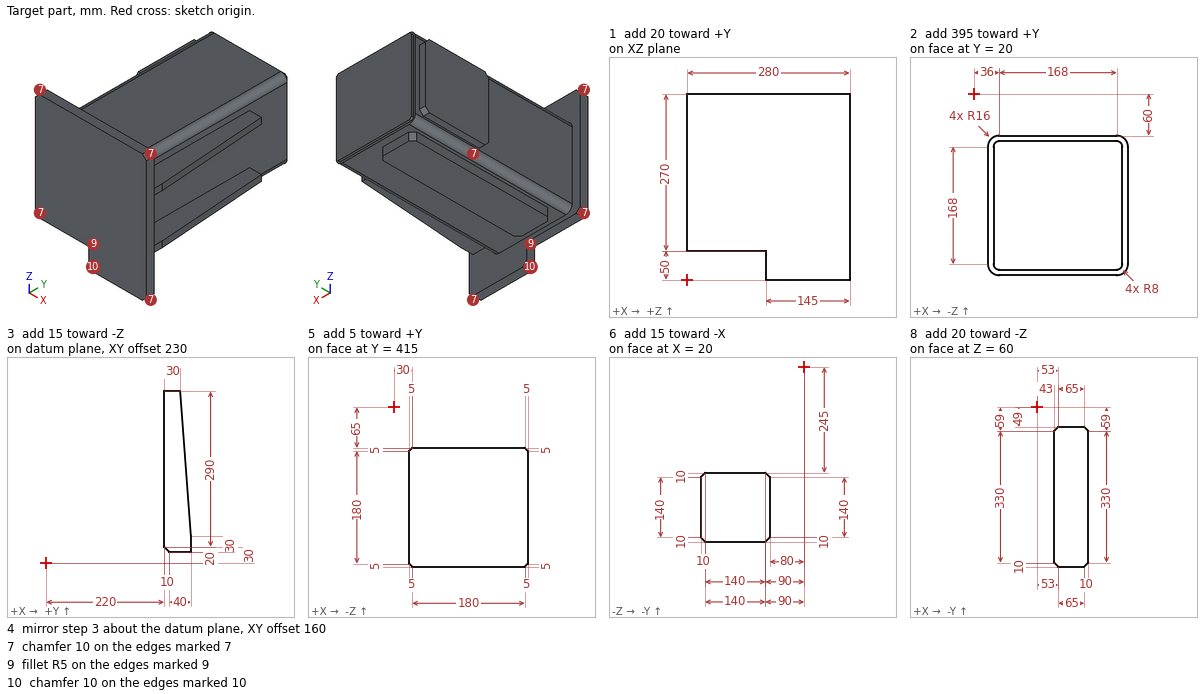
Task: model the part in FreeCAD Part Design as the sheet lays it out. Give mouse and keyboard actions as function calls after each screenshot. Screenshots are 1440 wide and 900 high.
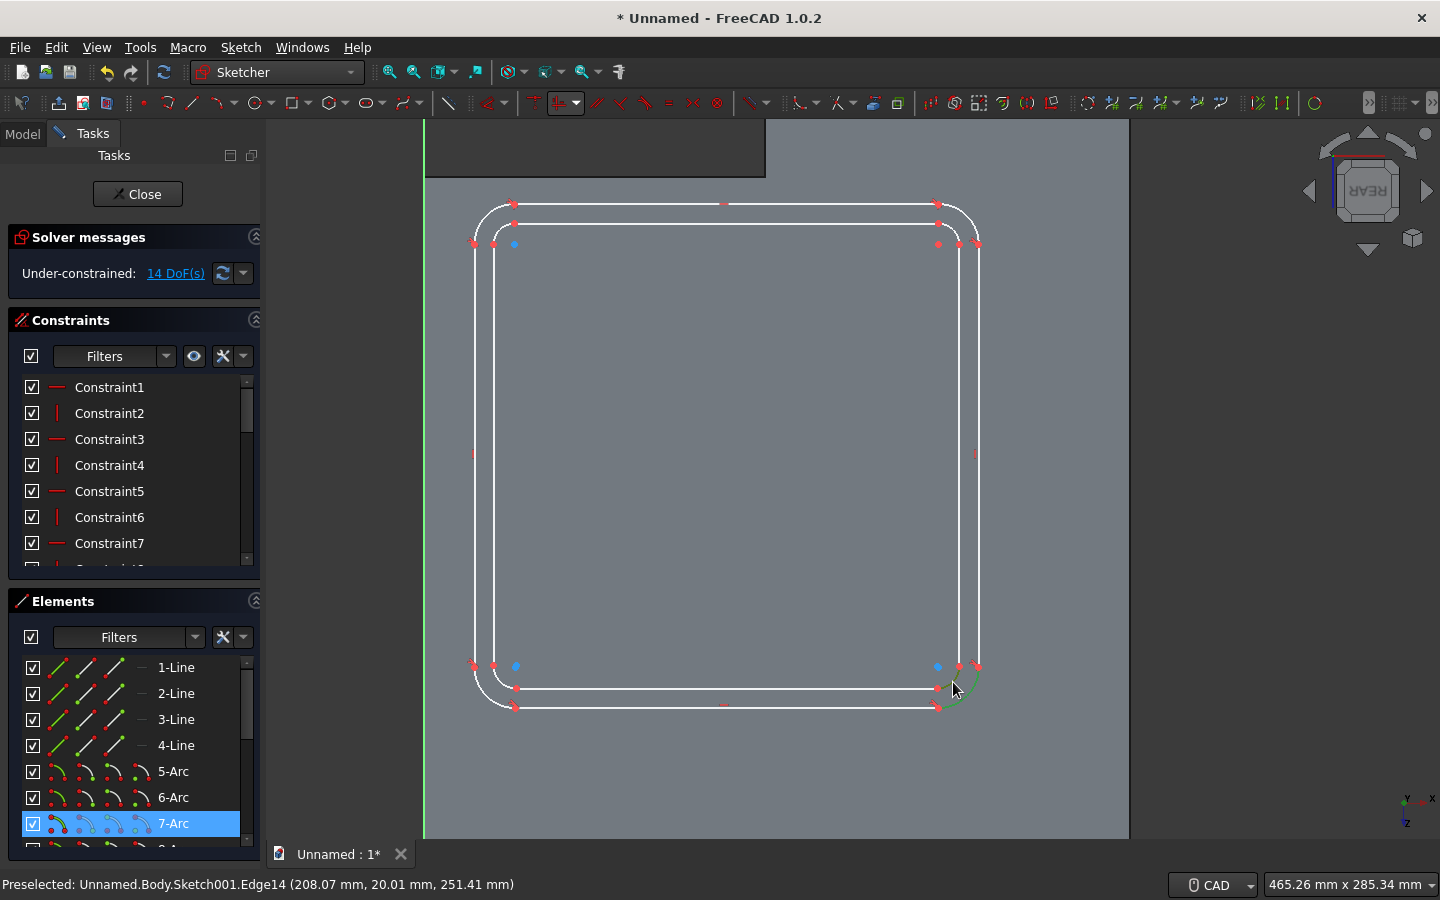
click(534, 104)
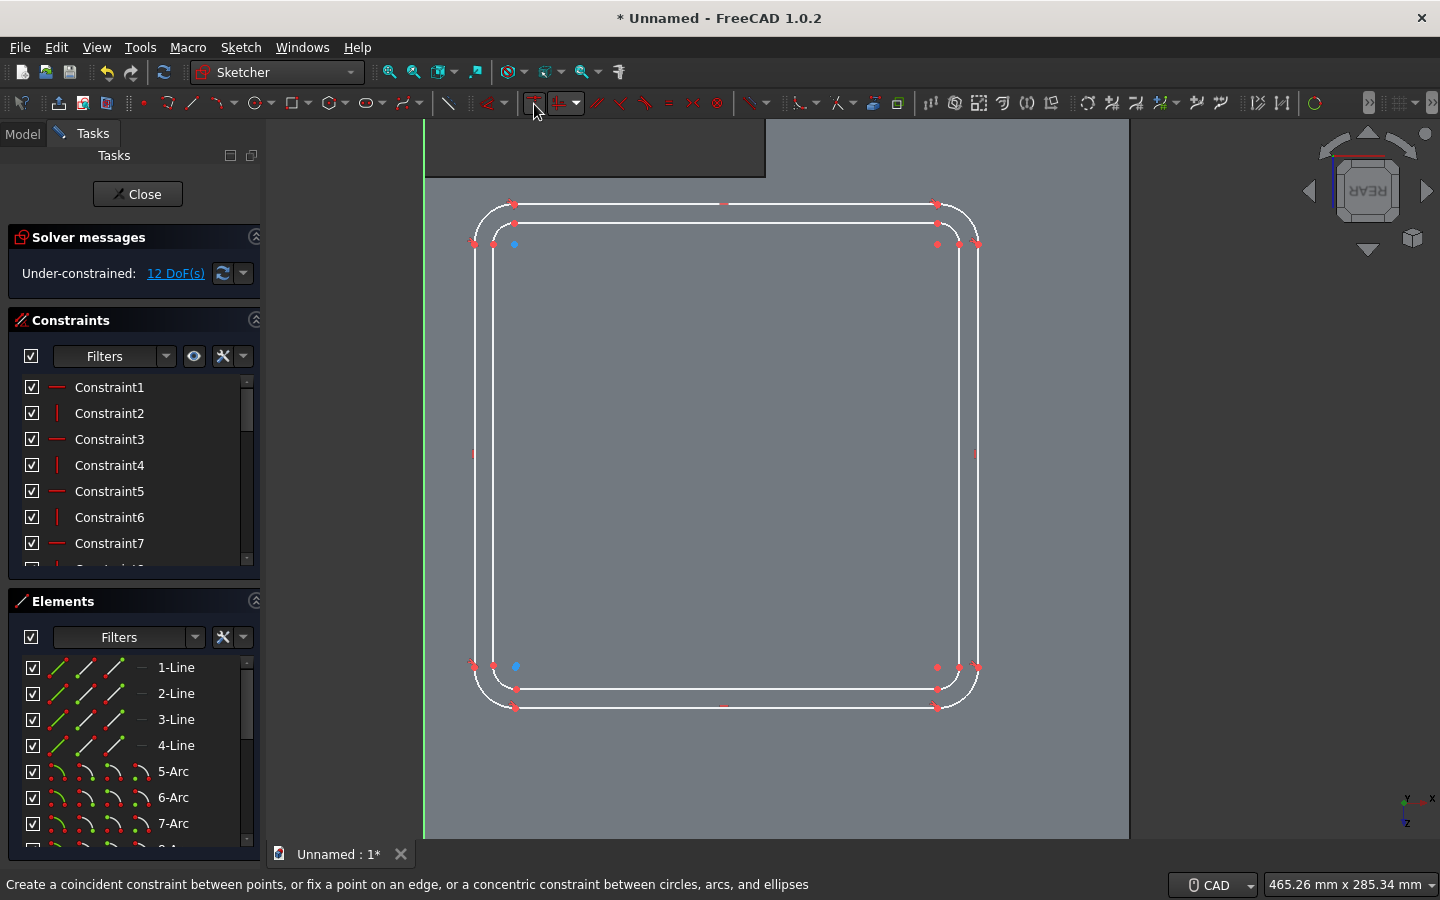
click(479, 686)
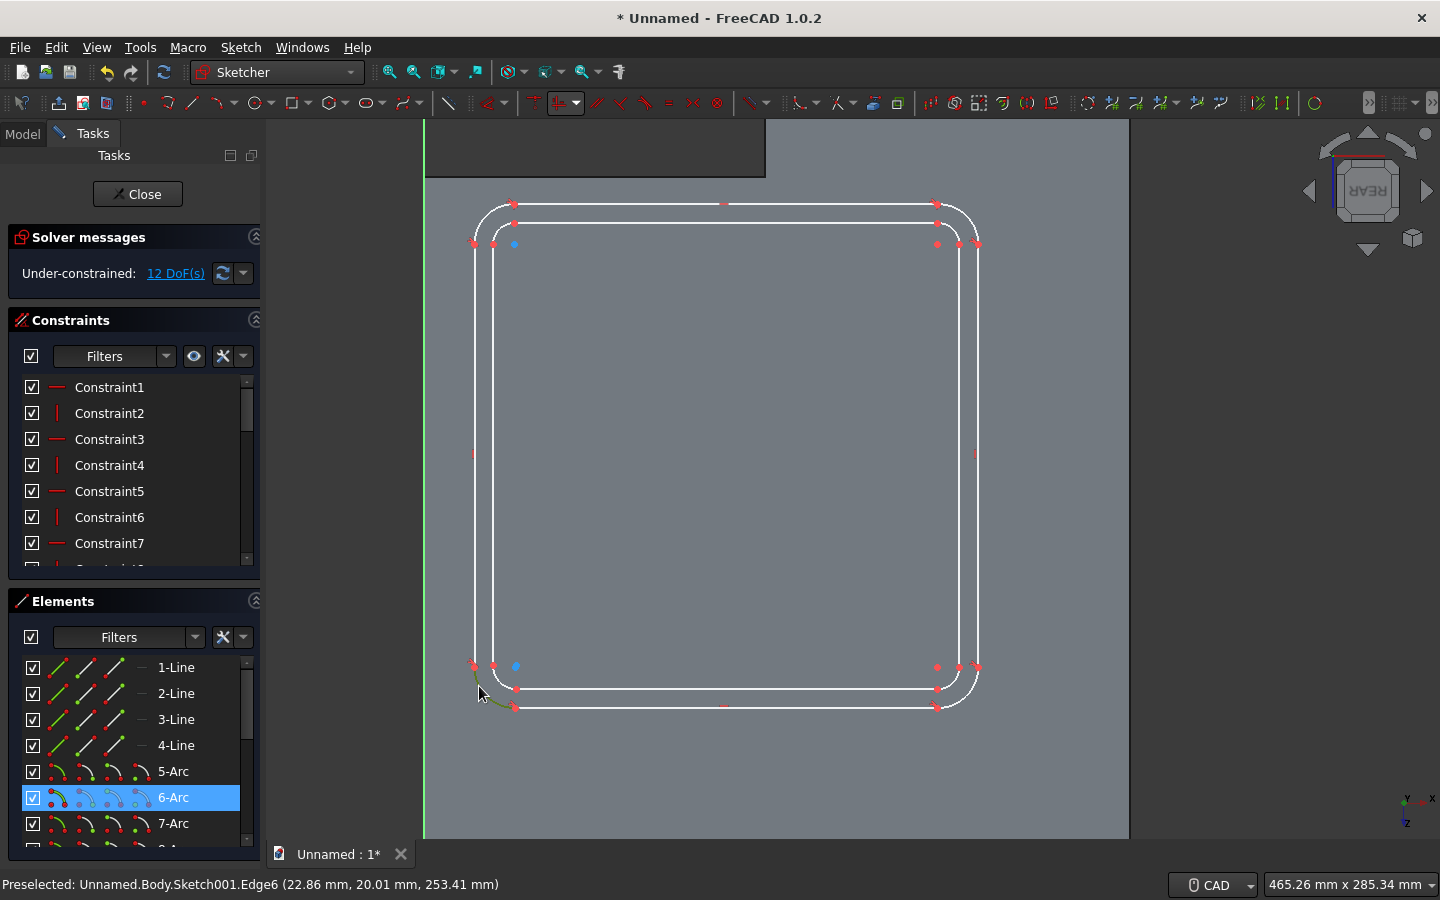
scroll(496, 676, up, 2)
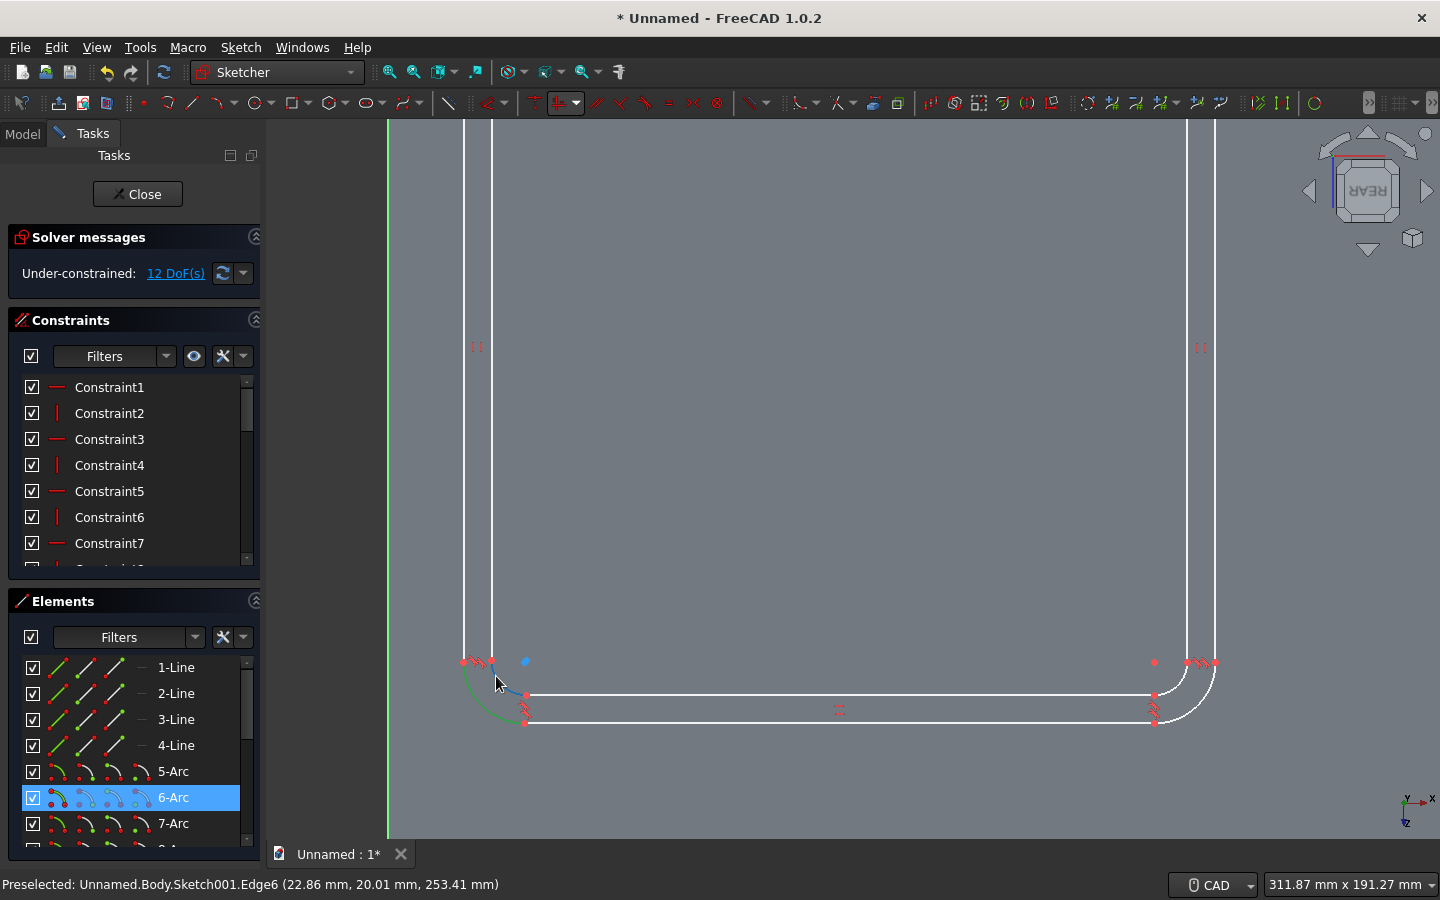
click(495, 676)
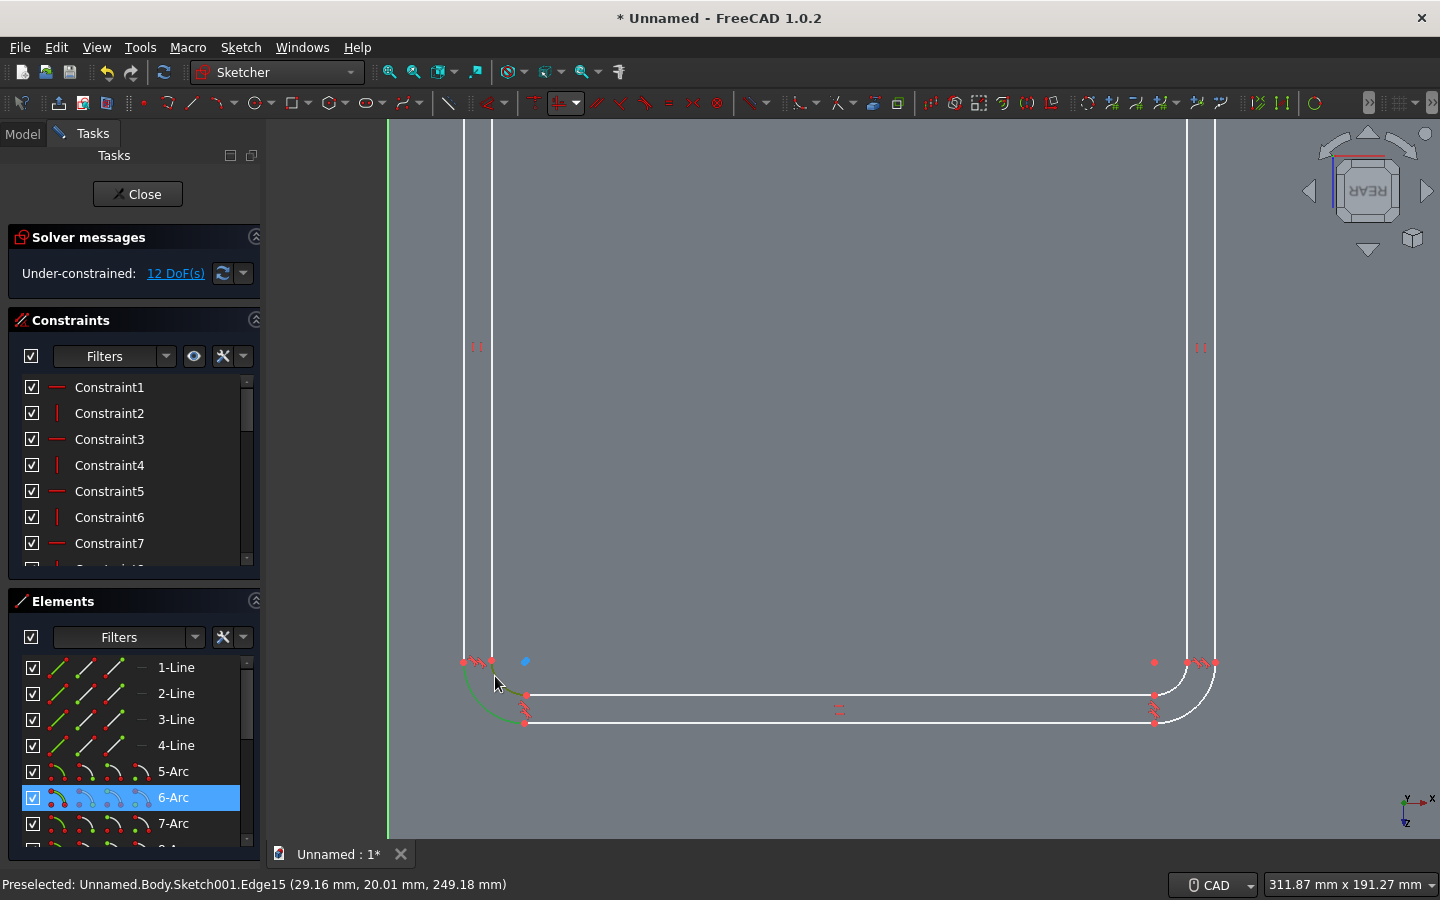
key(c)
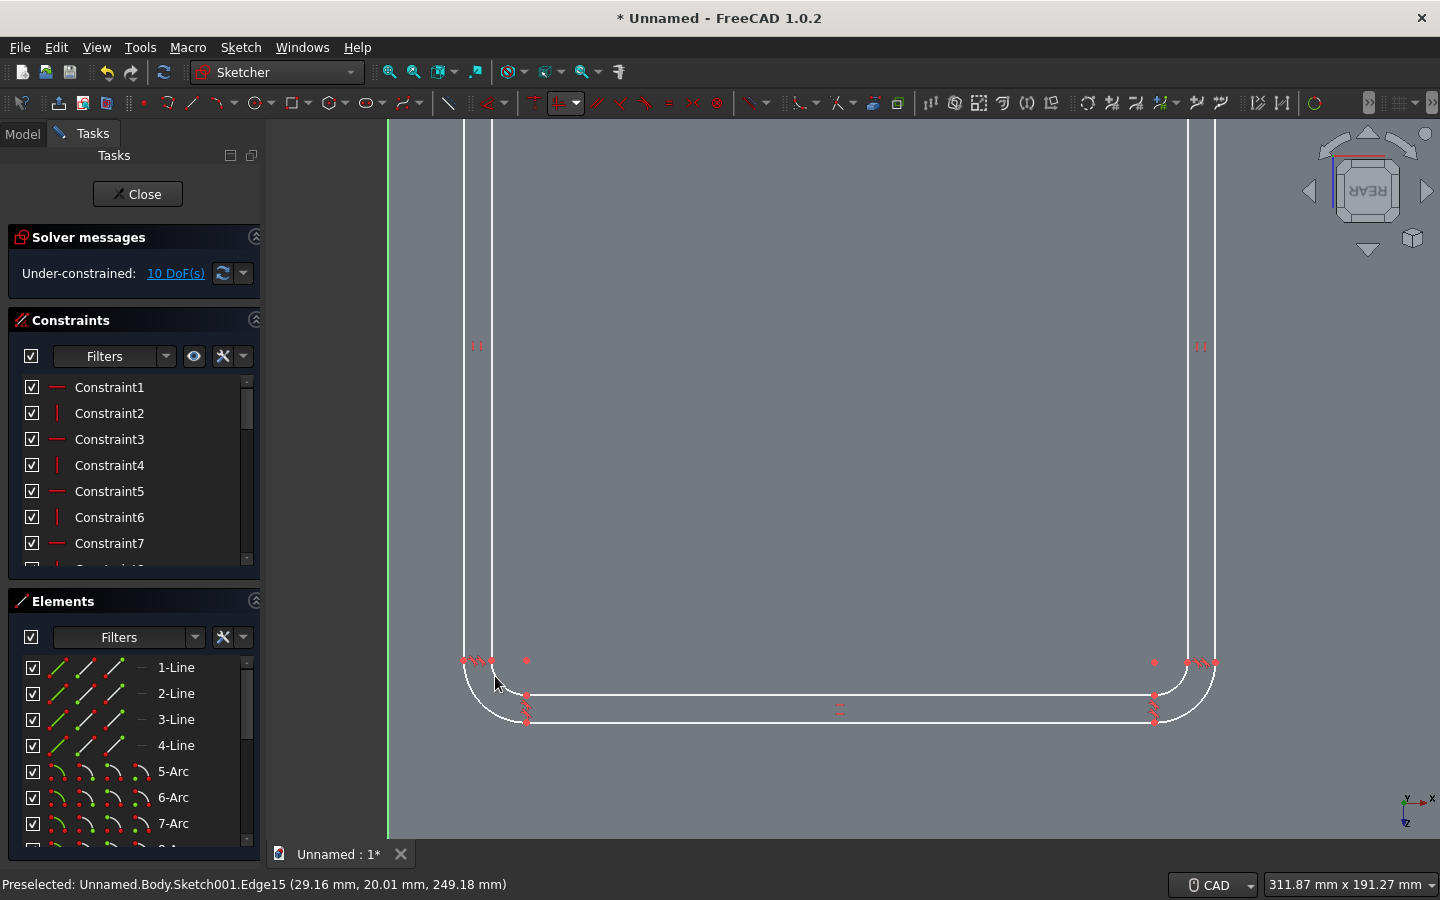
scroll(770, 680, down, 4)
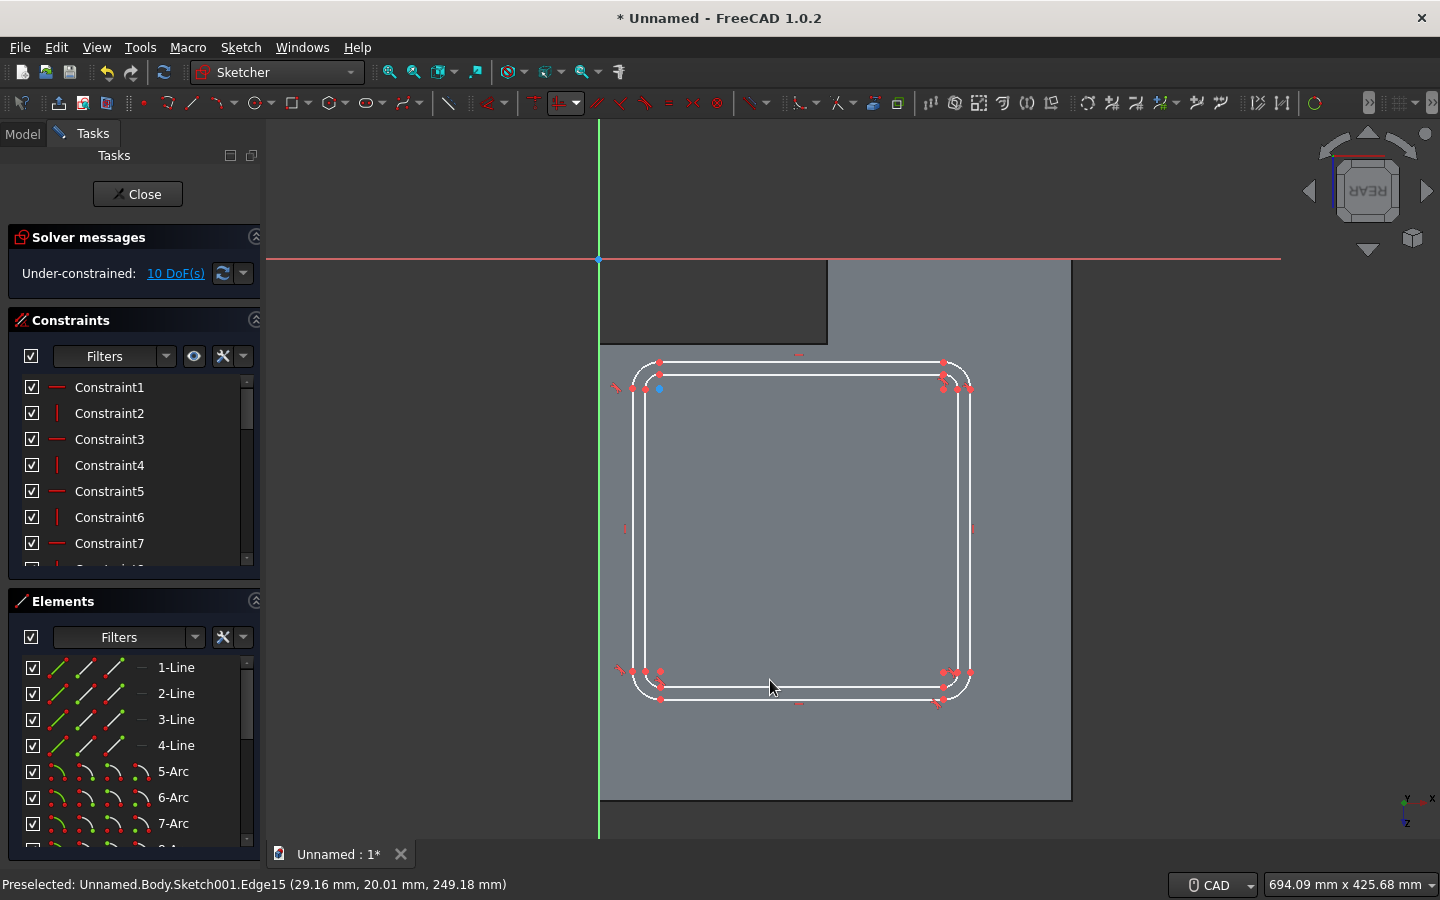
click(647, 365)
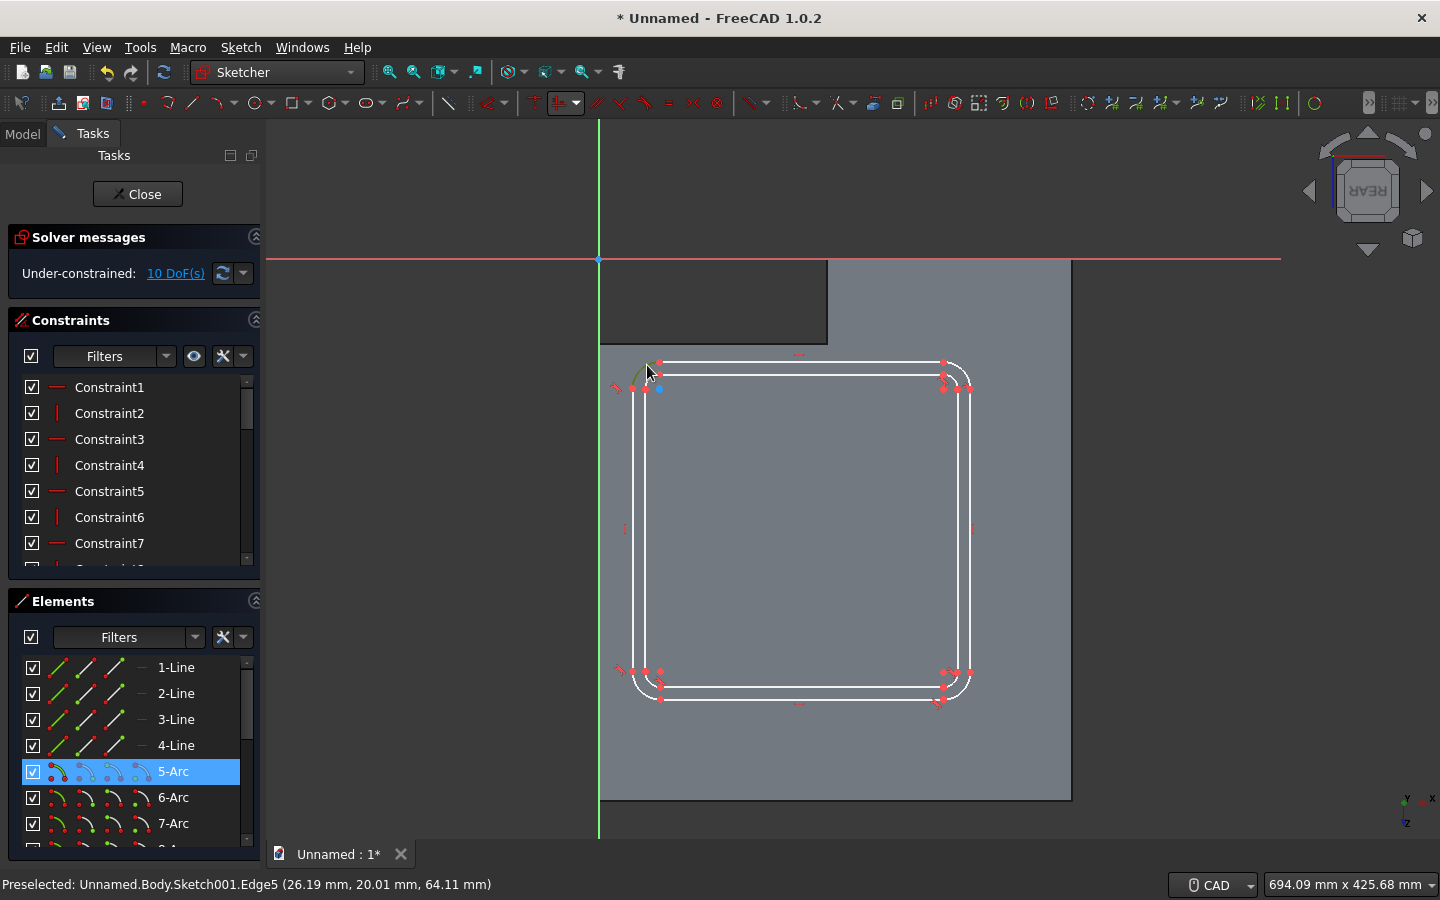
click(636, 684)